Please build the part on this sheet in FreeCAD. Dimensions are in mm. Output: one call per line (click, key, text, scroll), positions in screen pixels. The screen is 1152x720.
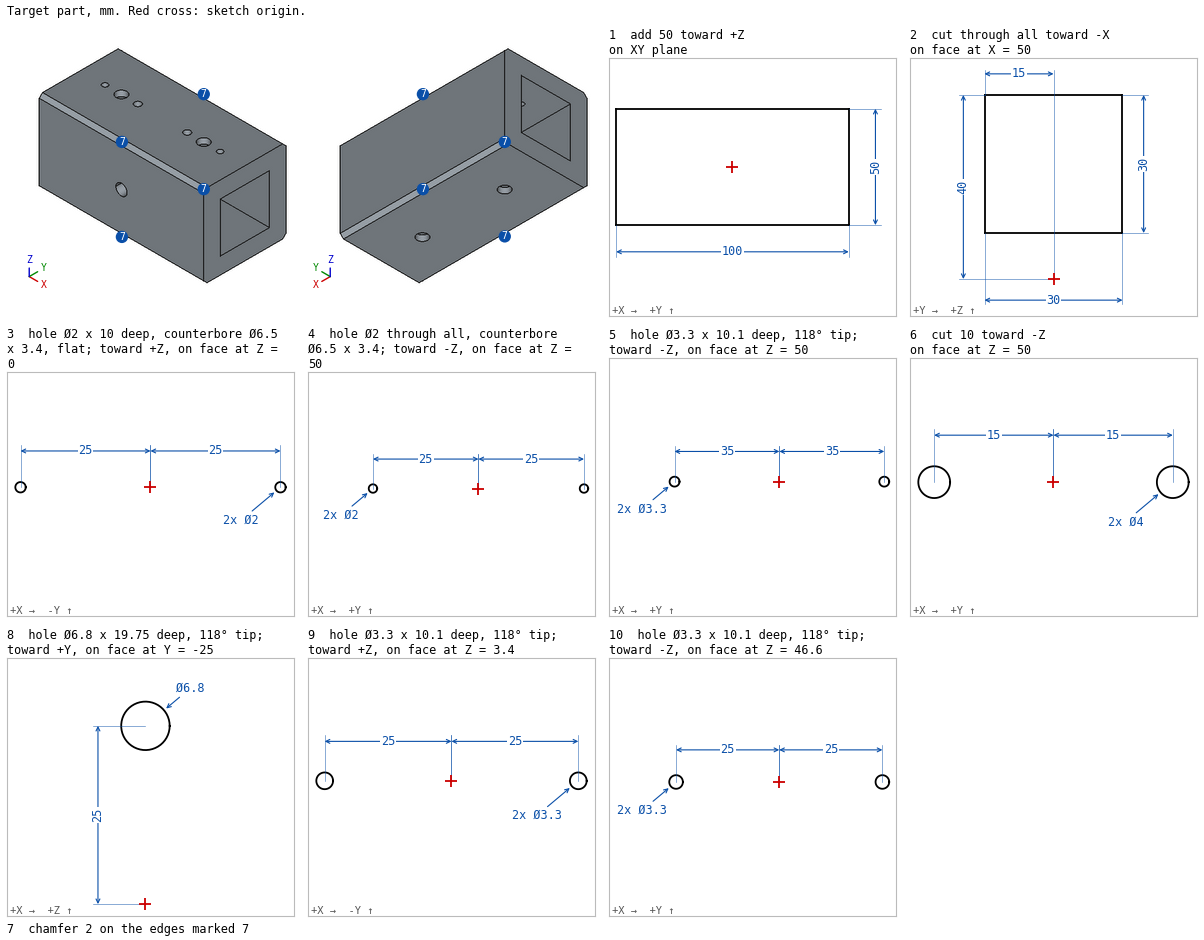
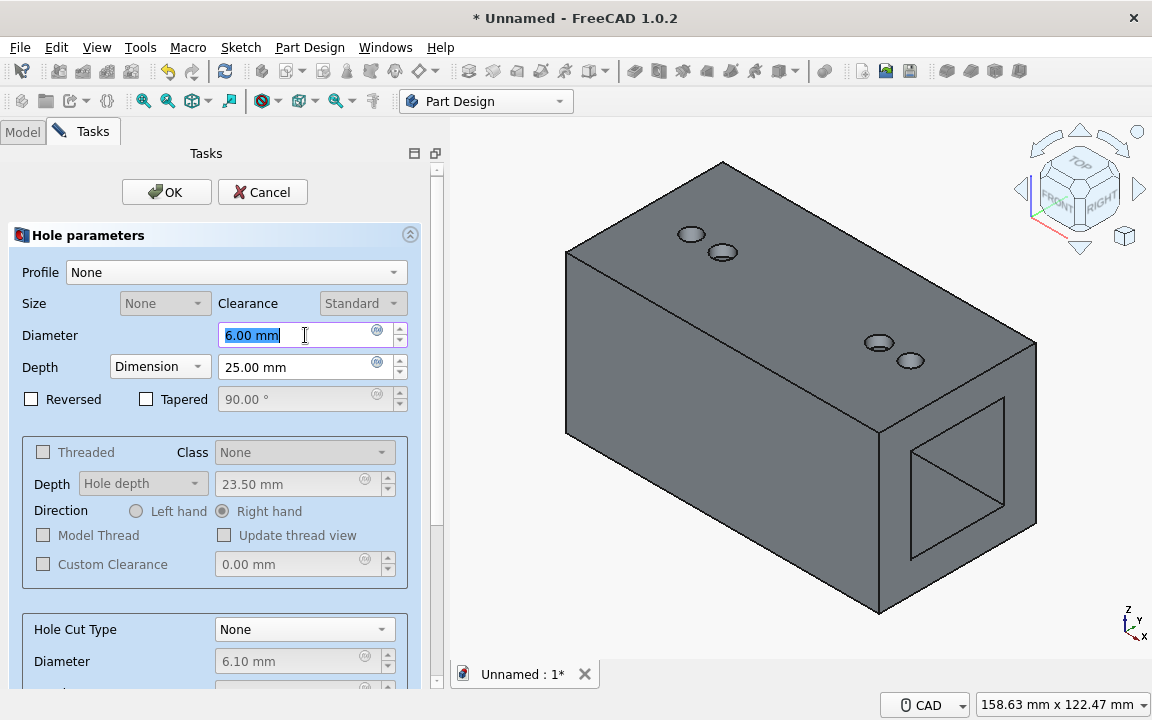
text(3.3)
key(Tab)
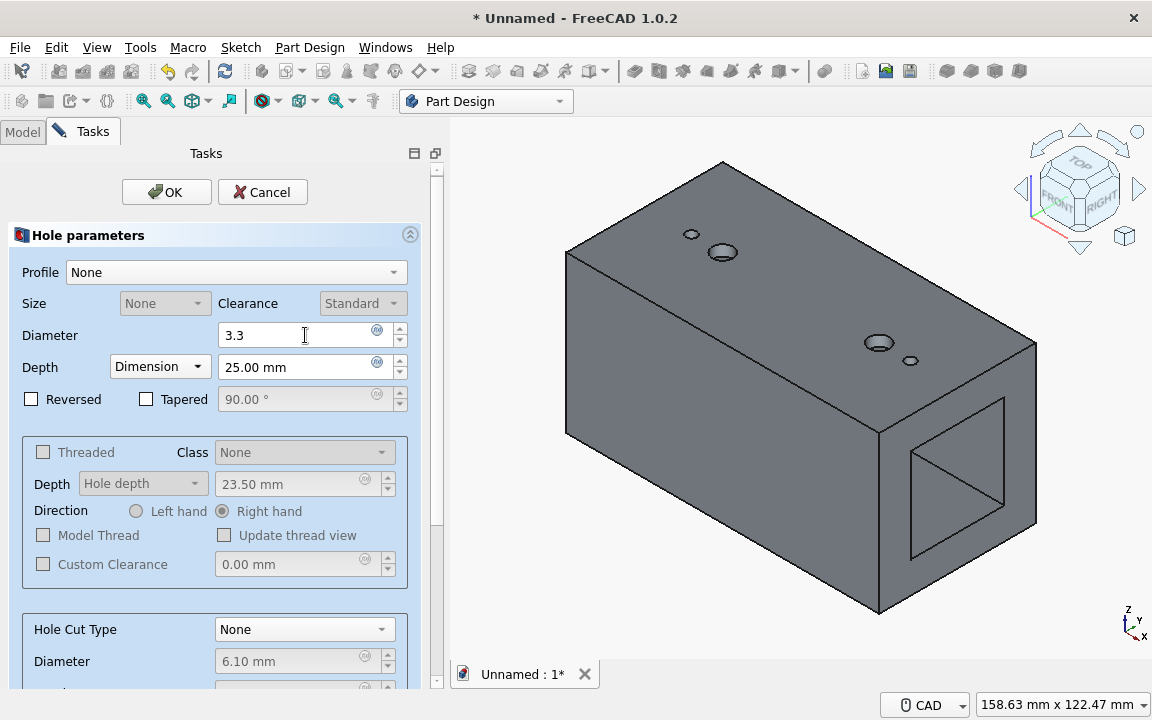
triple_click(305, 367)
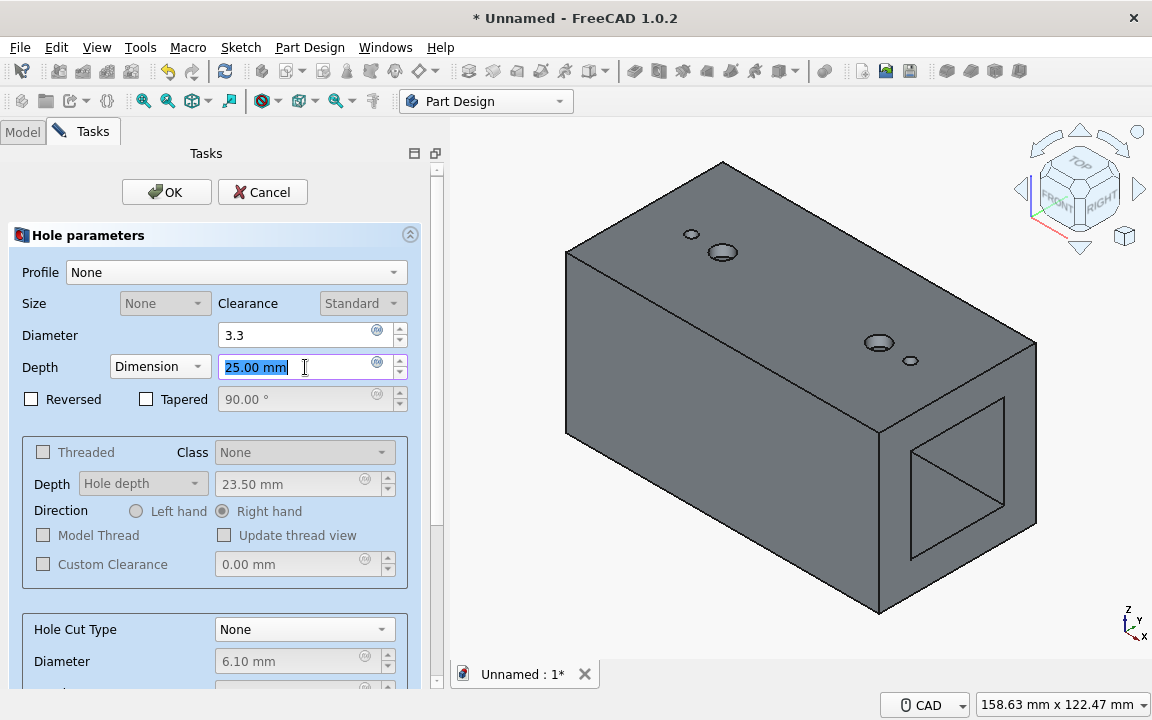
text(10.1)
key(Tab)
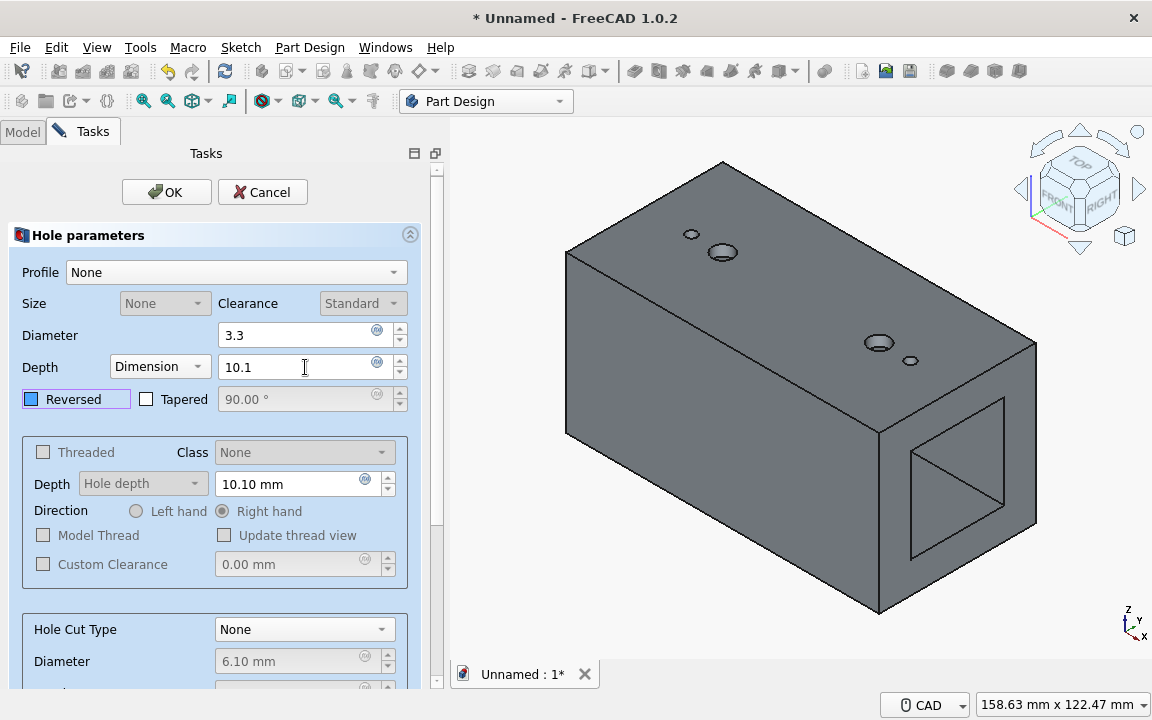
click(167, 192)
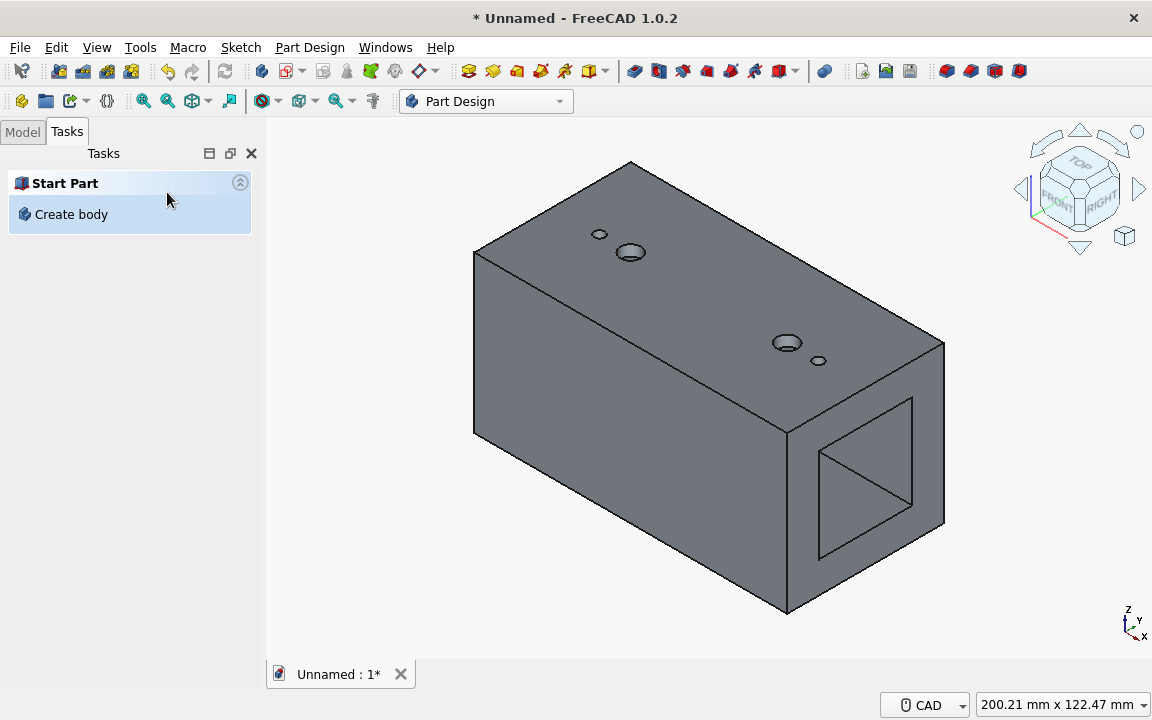
click(709, 297)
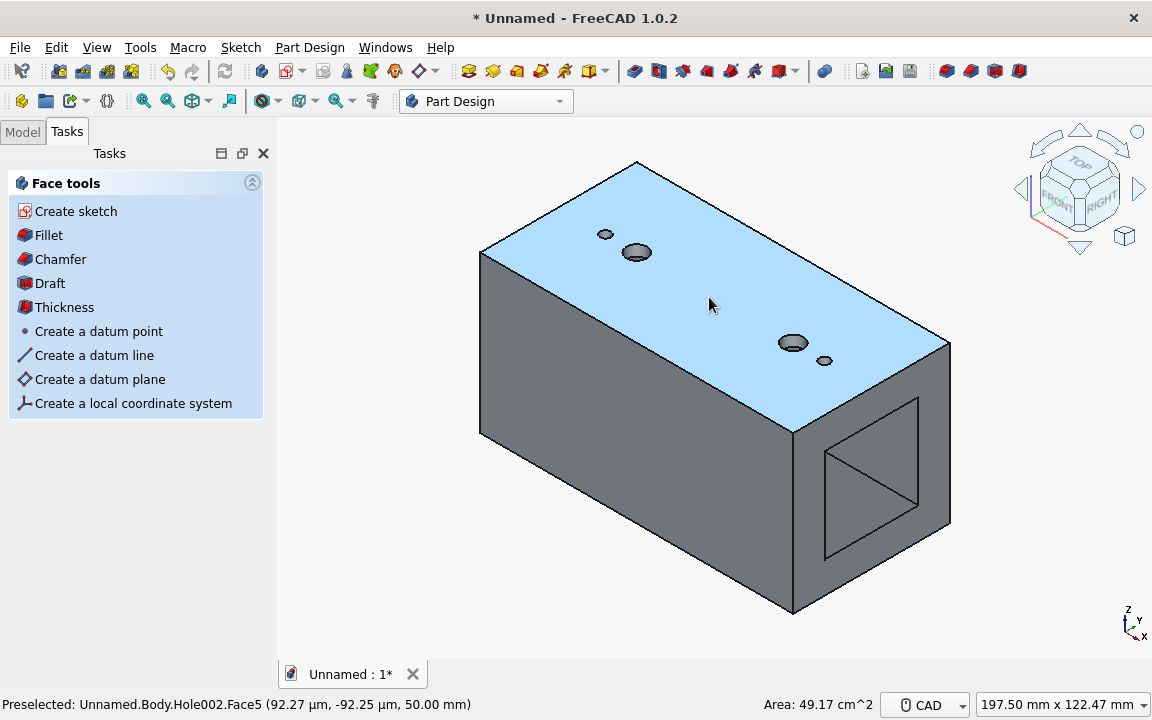
click(286, 72)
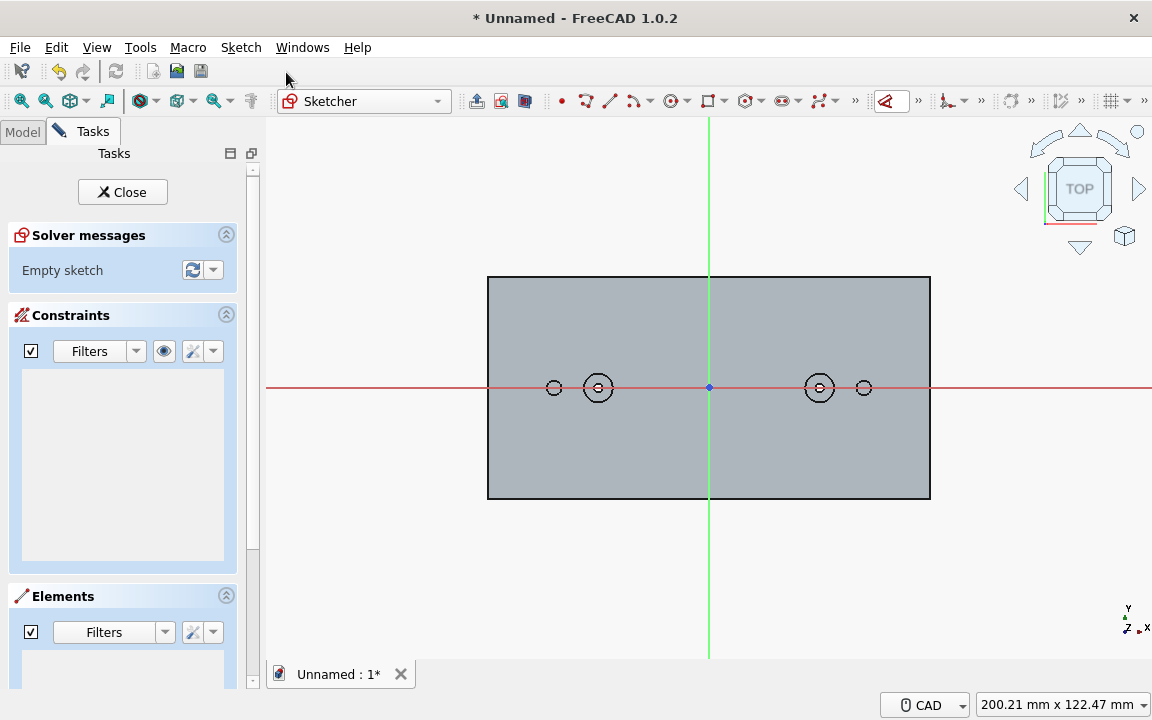
scroll(739, 388, up, 6)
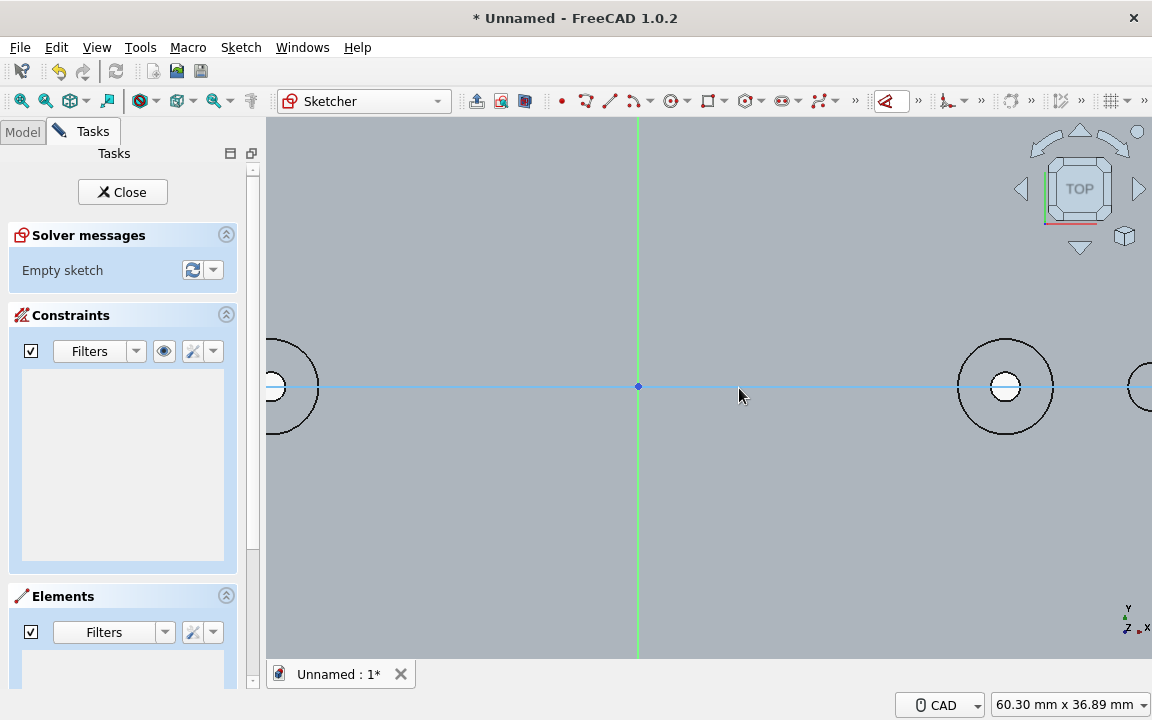
key(g)
key(c)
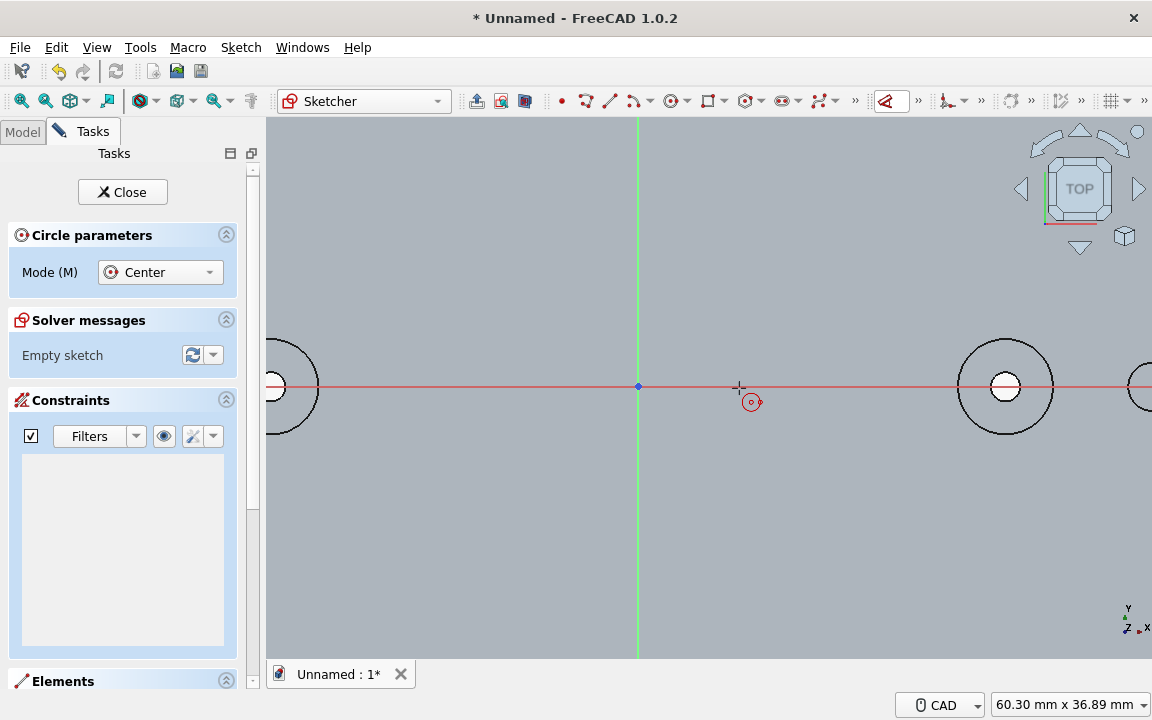
click(859, 387)
move(879, 366)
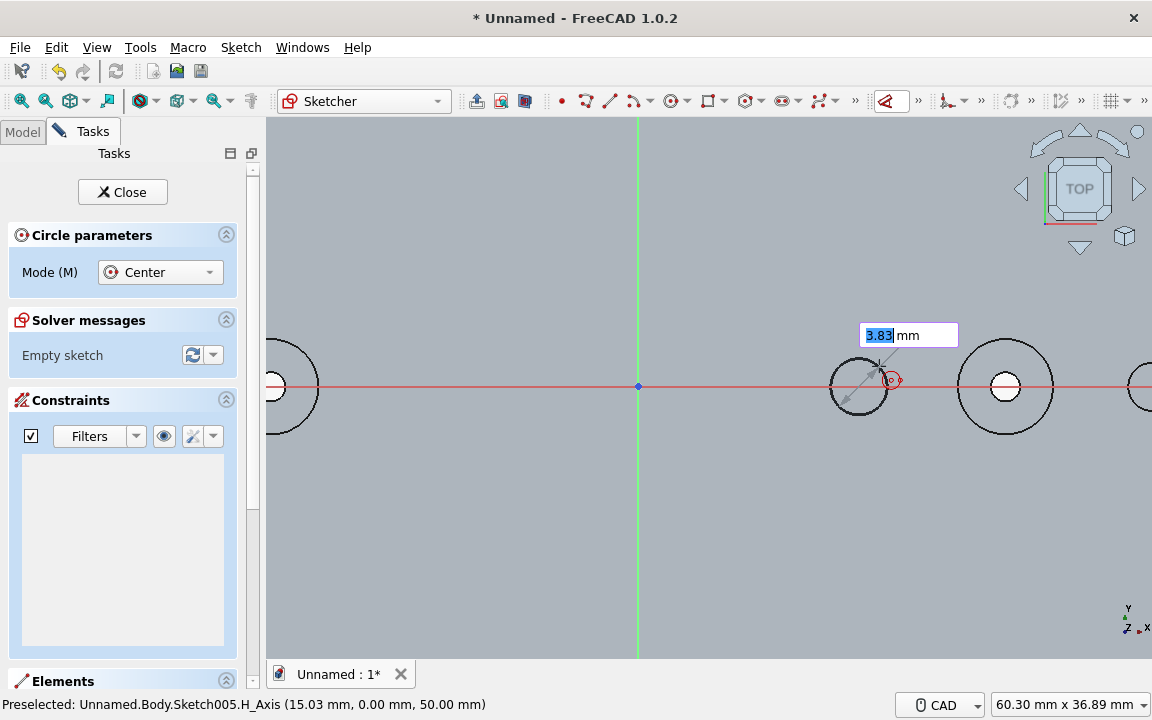
text(4)
key(Return)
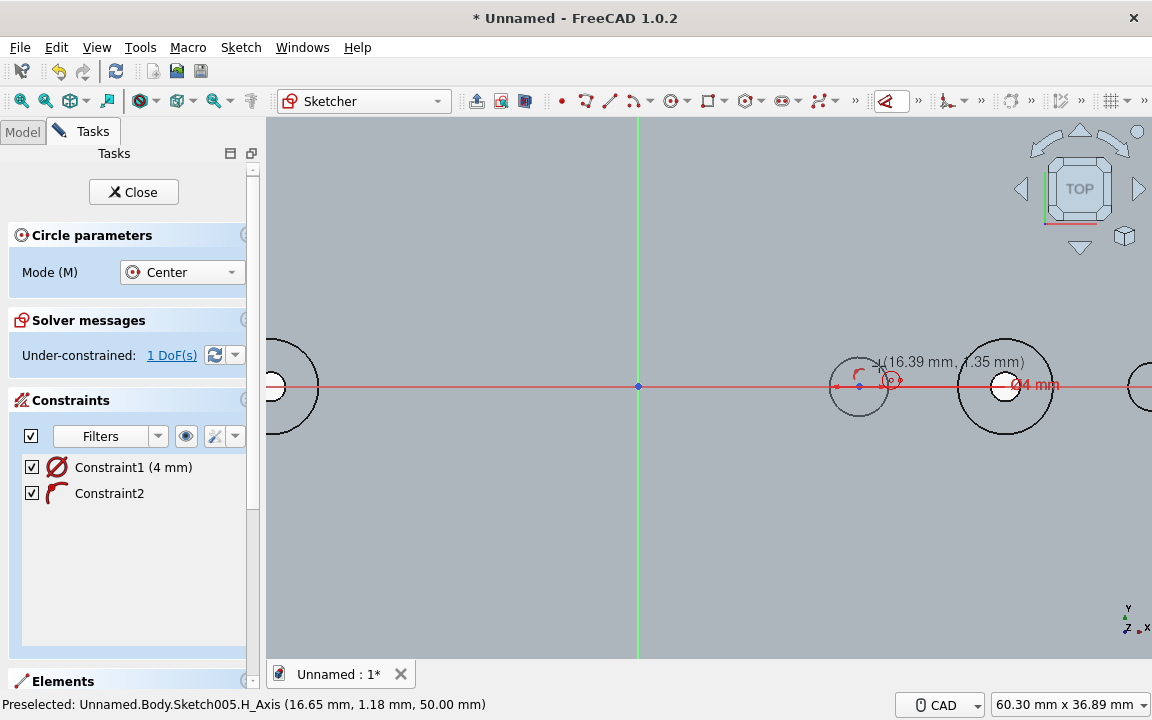
click(418, 387)
move(439, 366)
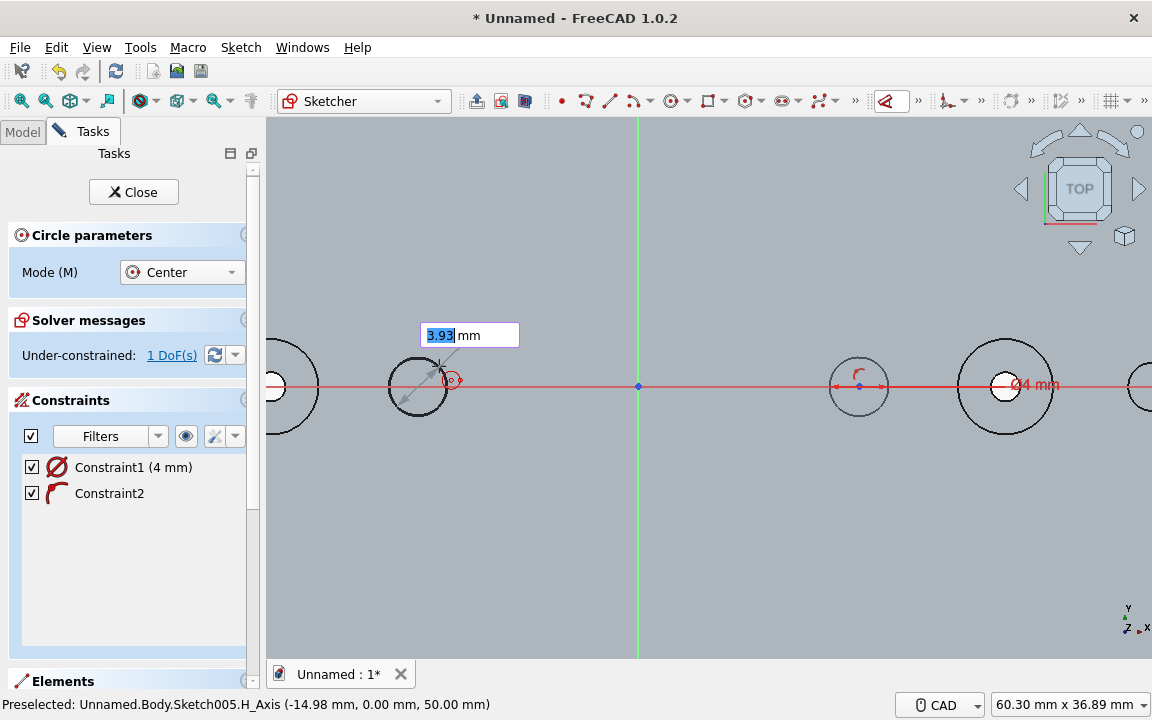
text(4)
key(Return)
key(Escape)